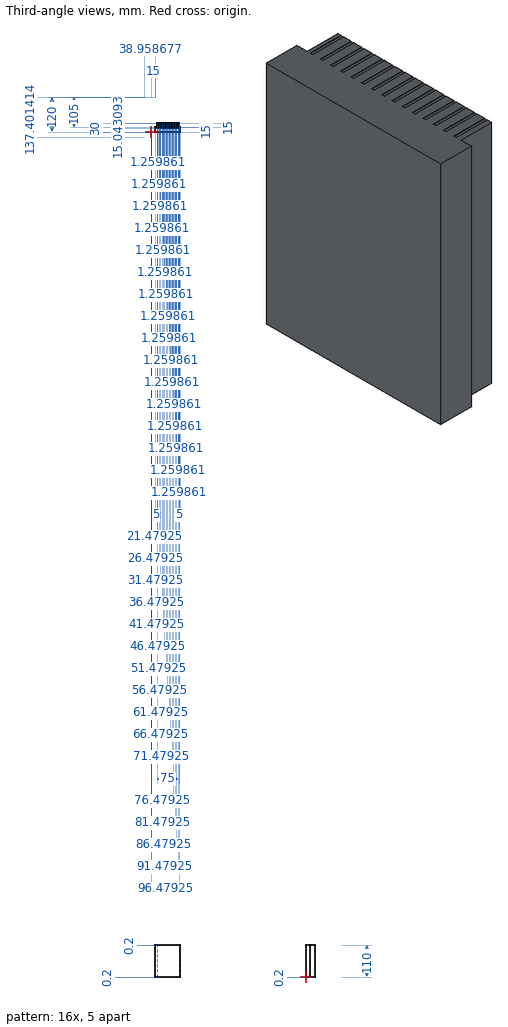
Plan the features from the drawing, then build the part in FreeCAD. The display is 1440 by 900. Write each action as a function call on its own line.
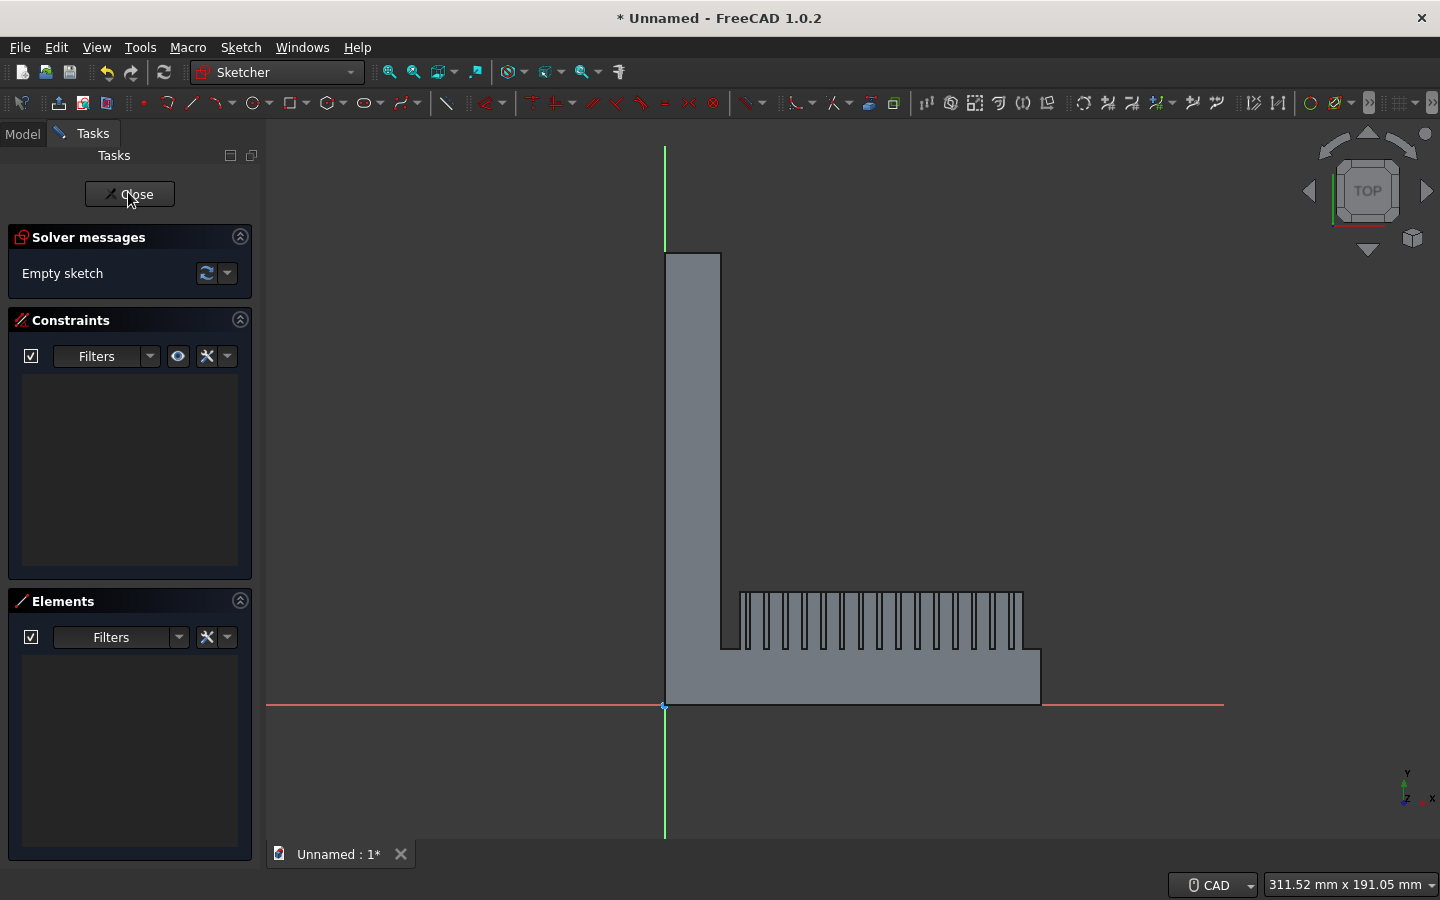
click(108, 104)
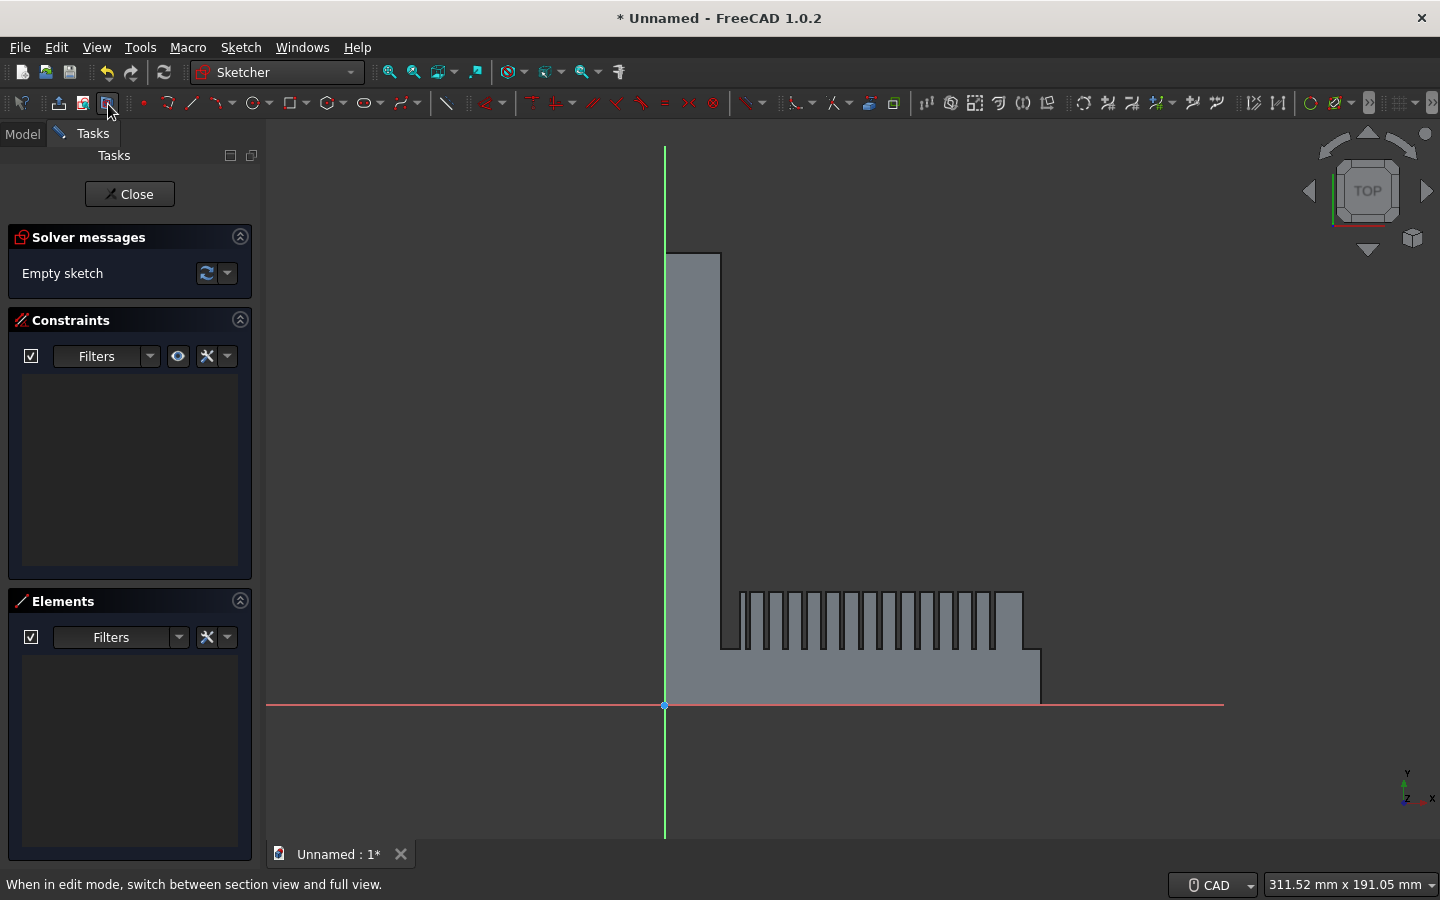
scroll(1040, 638, up, 11)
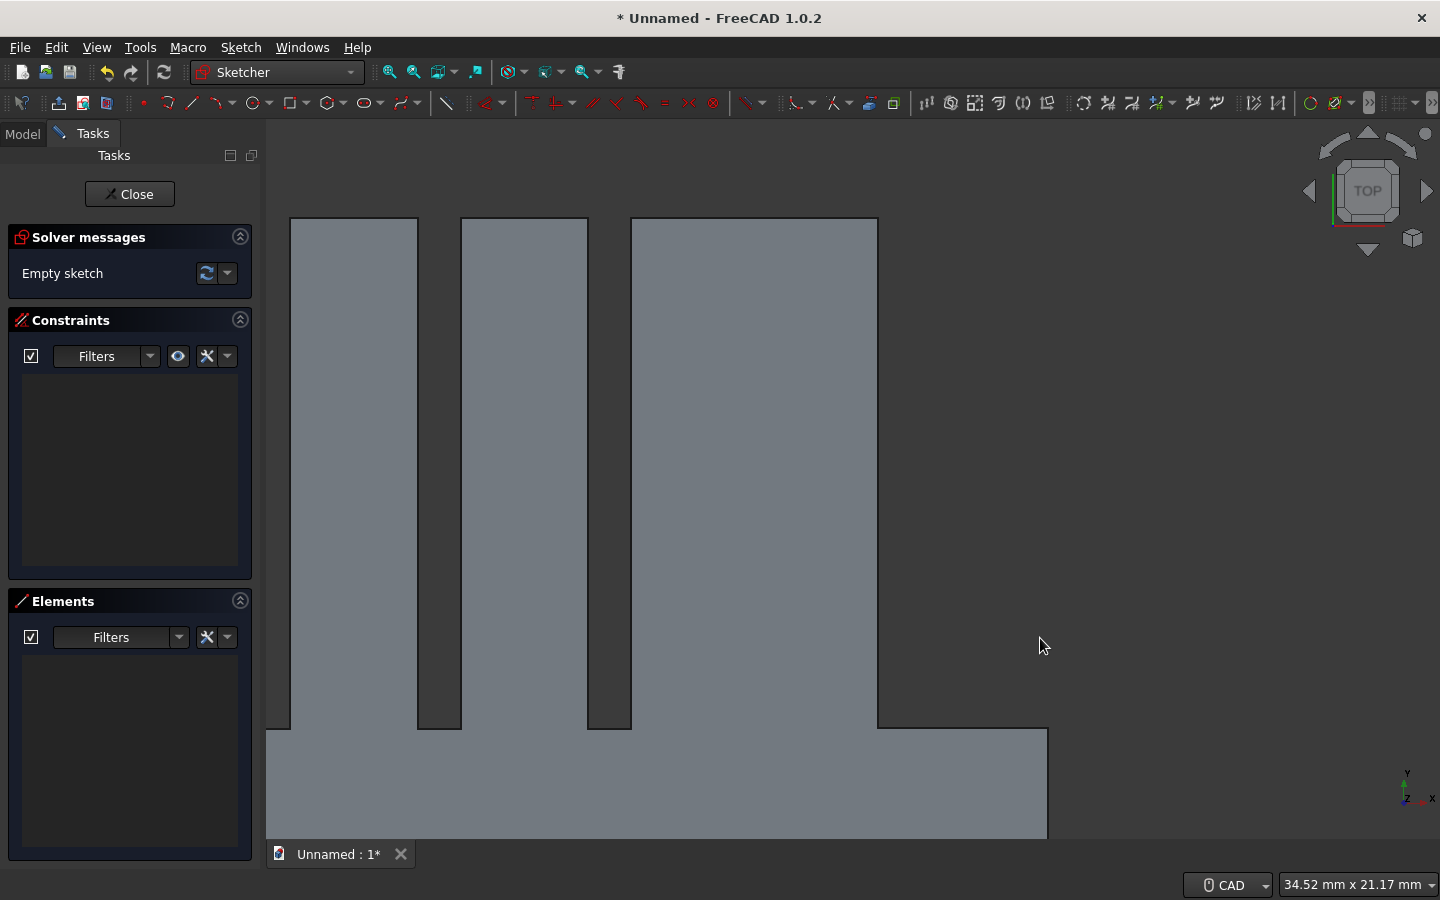
click(290, 104)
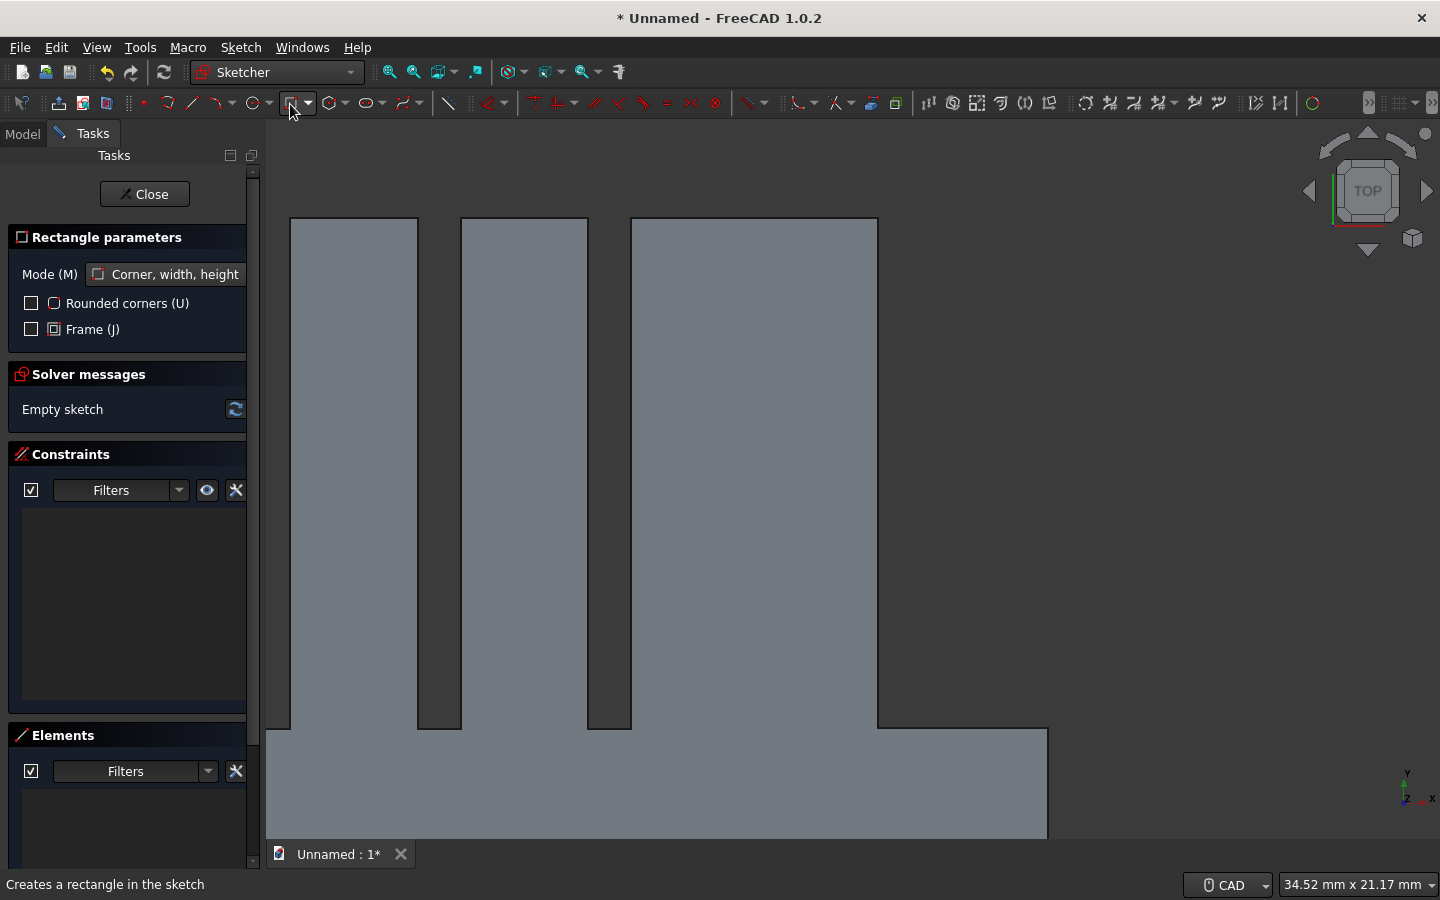
click(758, 218)
click(801, 729)
key(Escape)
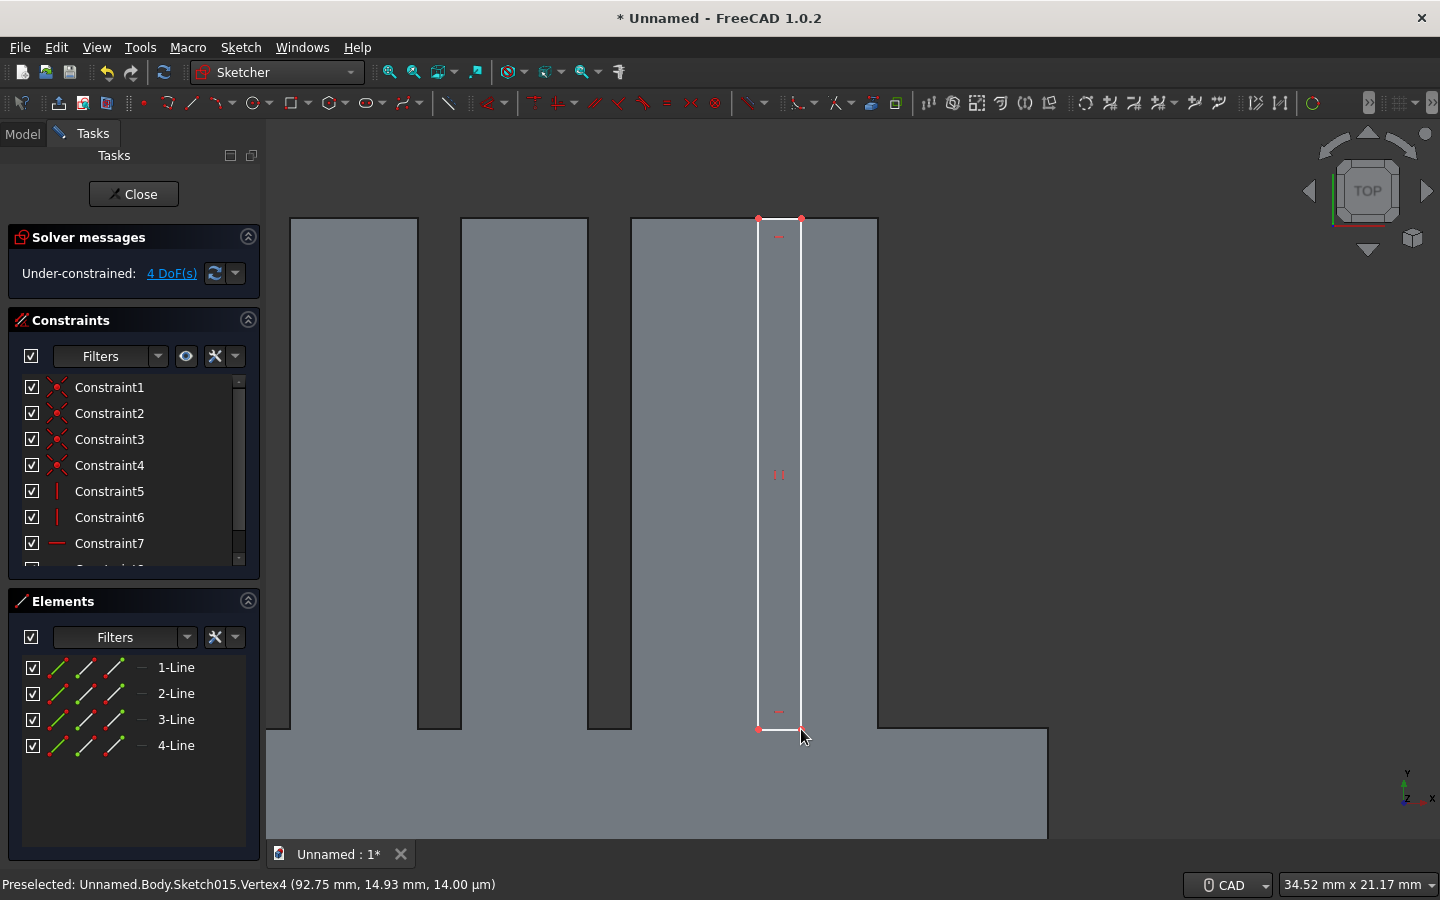
click(488, 104)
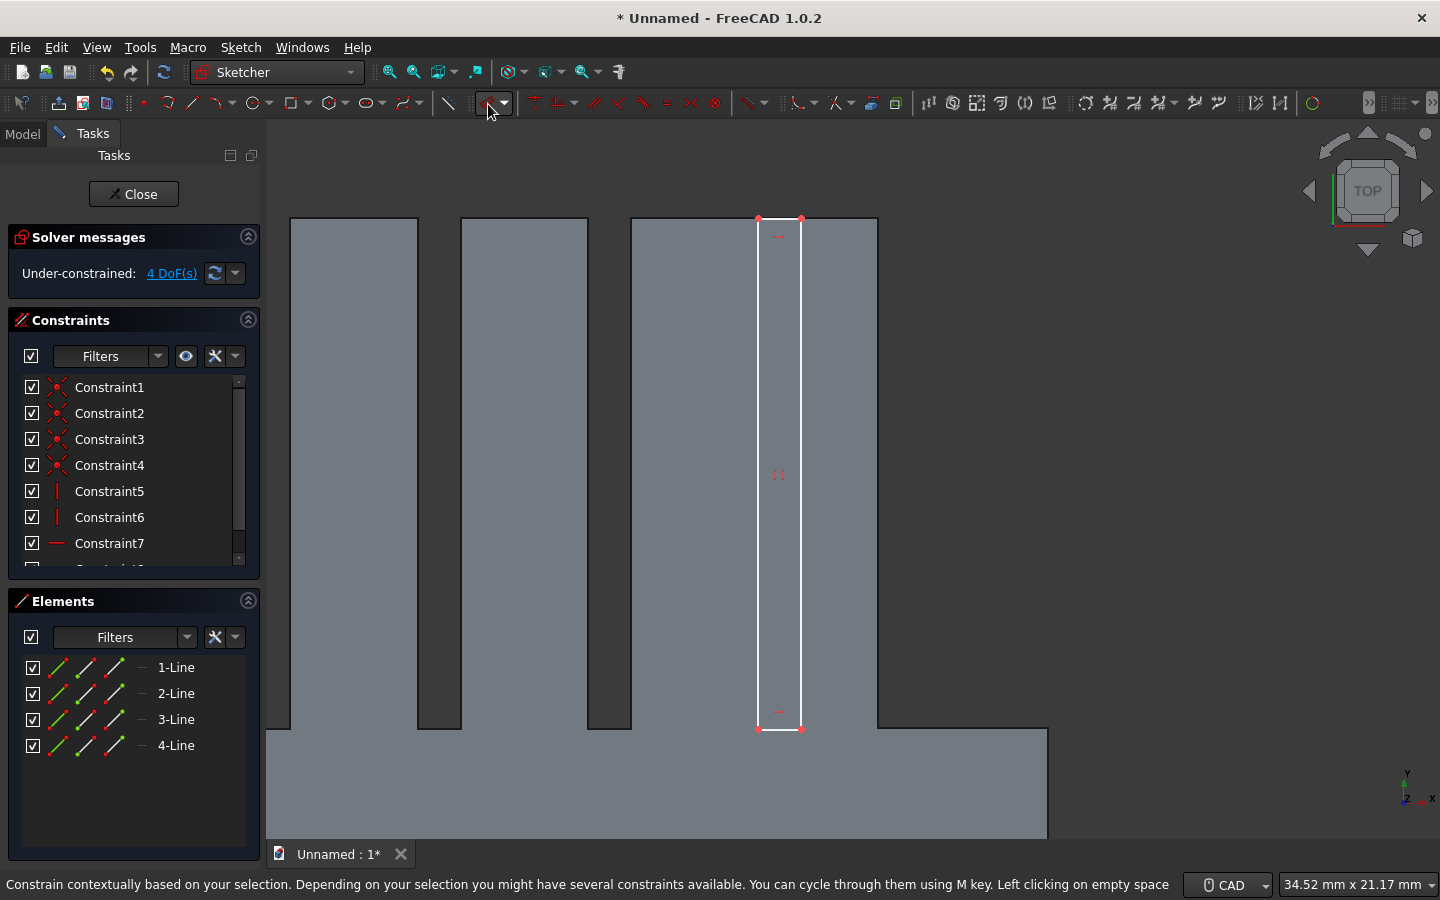
click(758, 219)
click(816, 515)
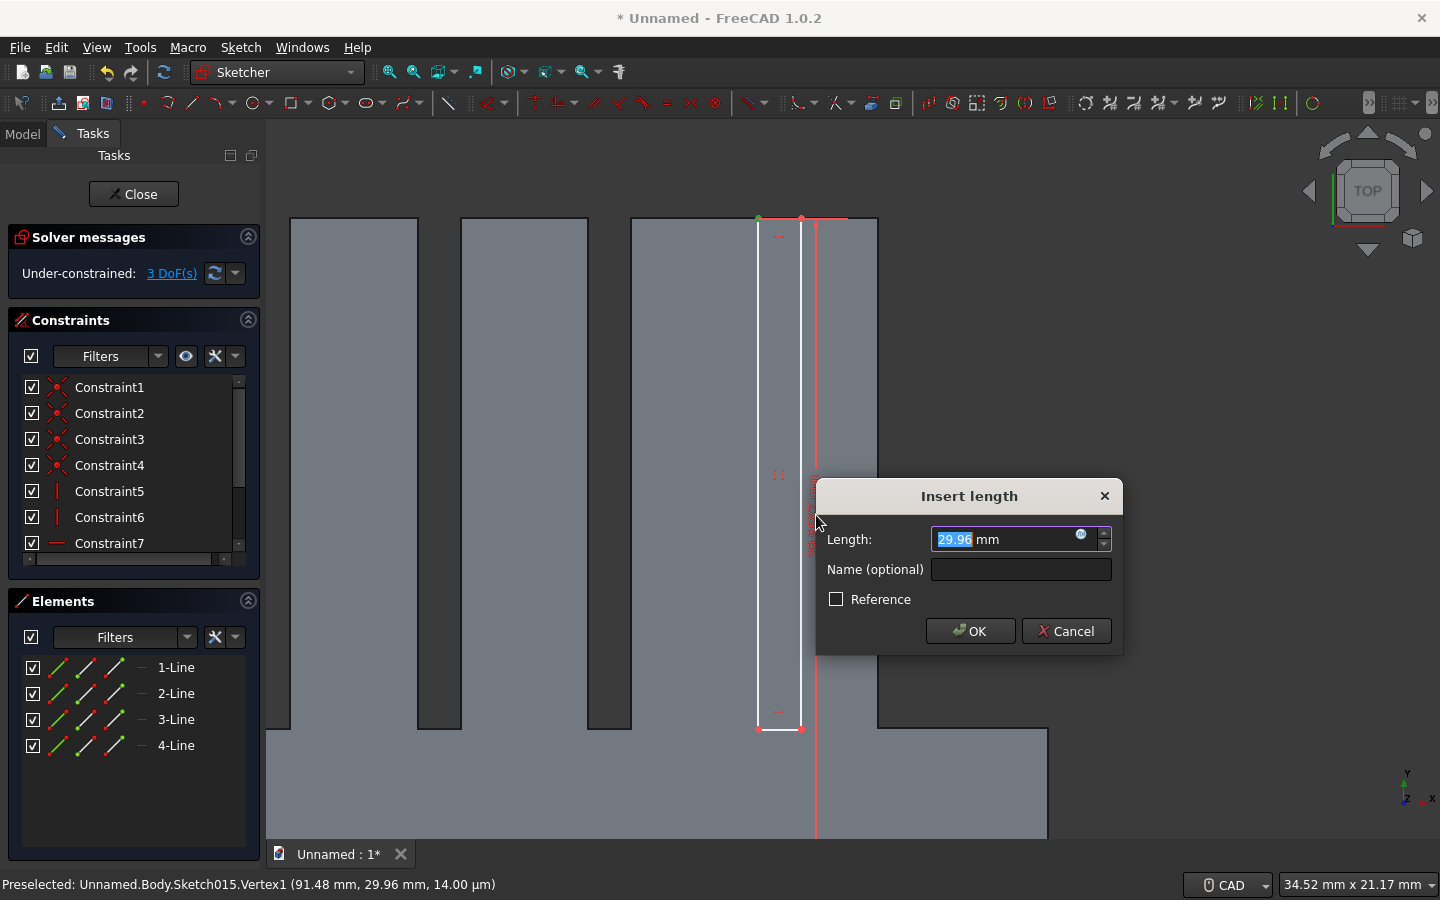
text(30)
key(Return)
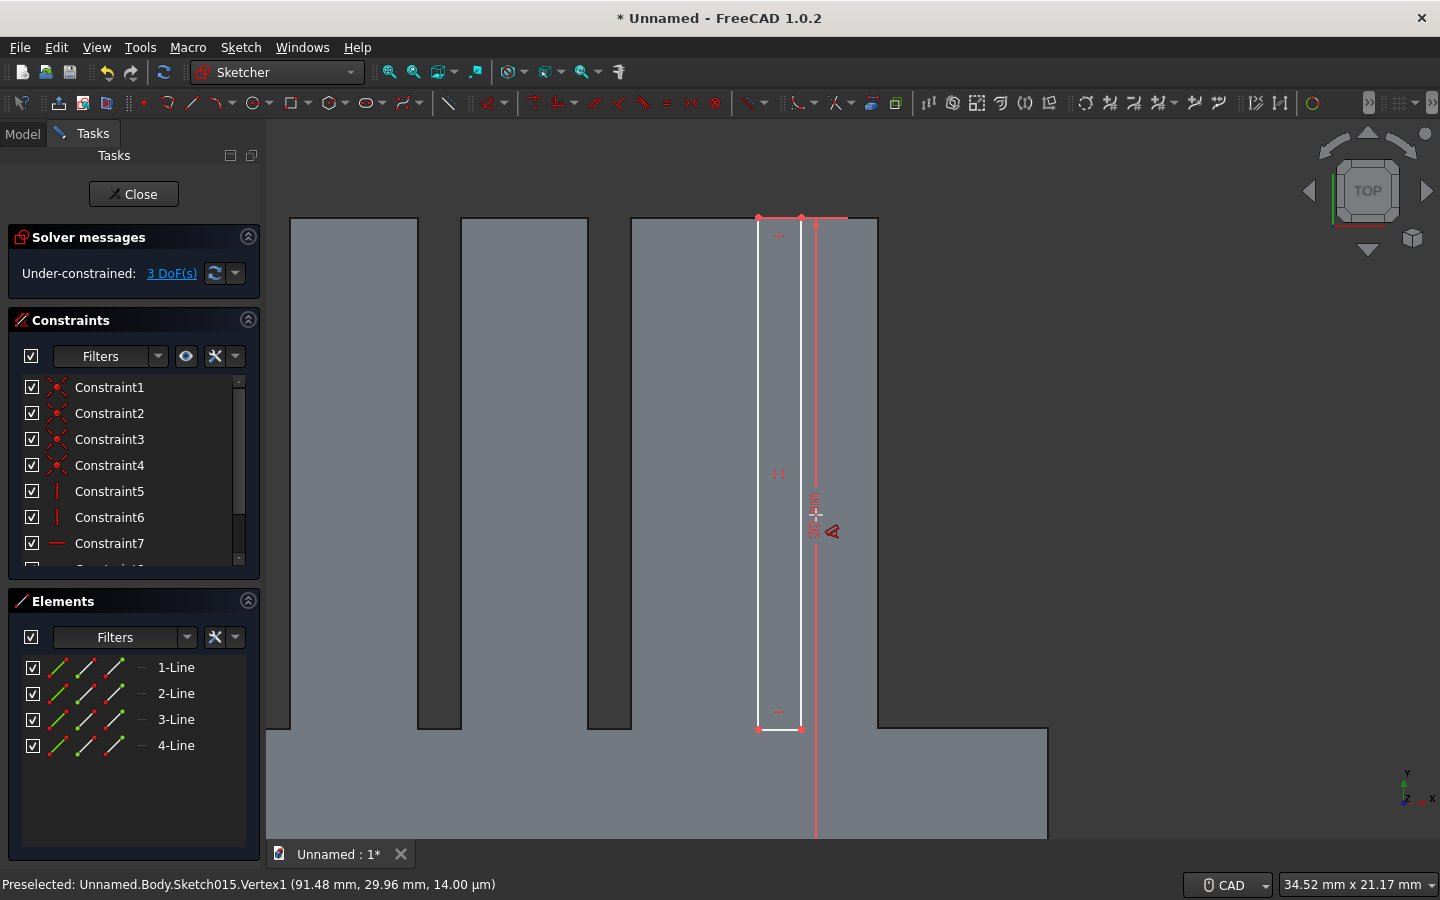
click(771, 730)
click(779, 764)